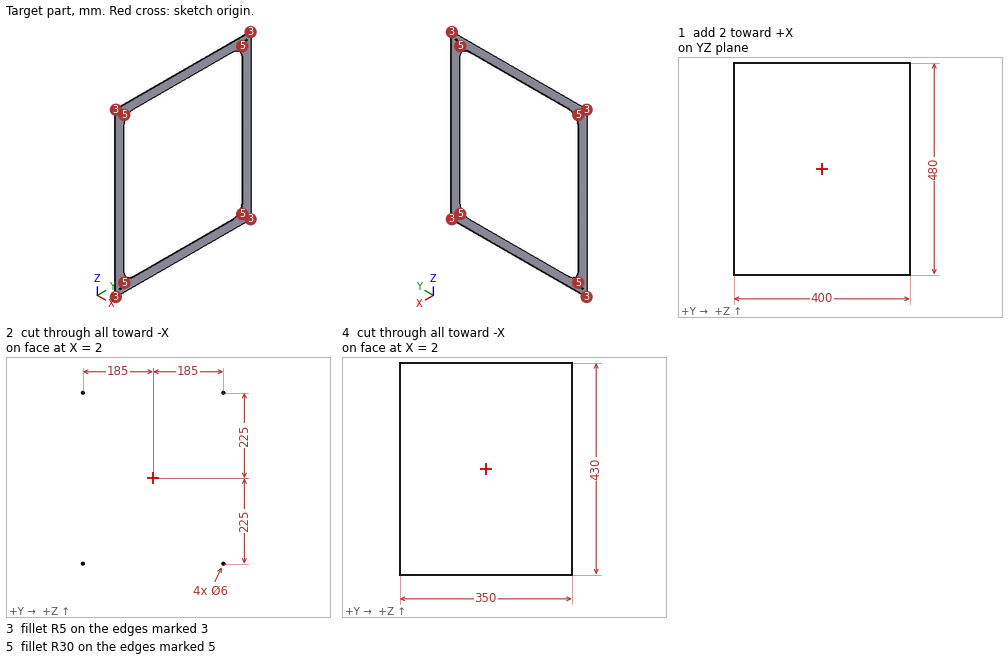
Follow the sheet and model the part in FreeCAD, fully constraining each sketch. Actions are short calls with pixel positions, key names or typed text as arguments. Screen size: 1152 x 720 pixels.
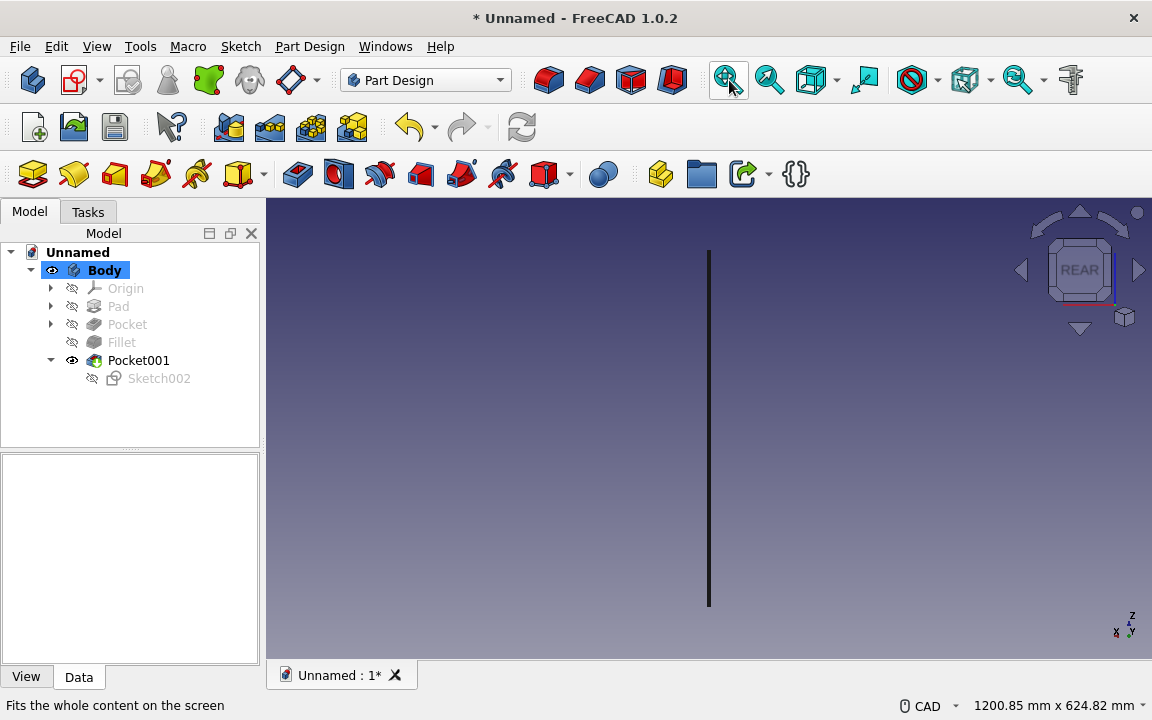
key(6)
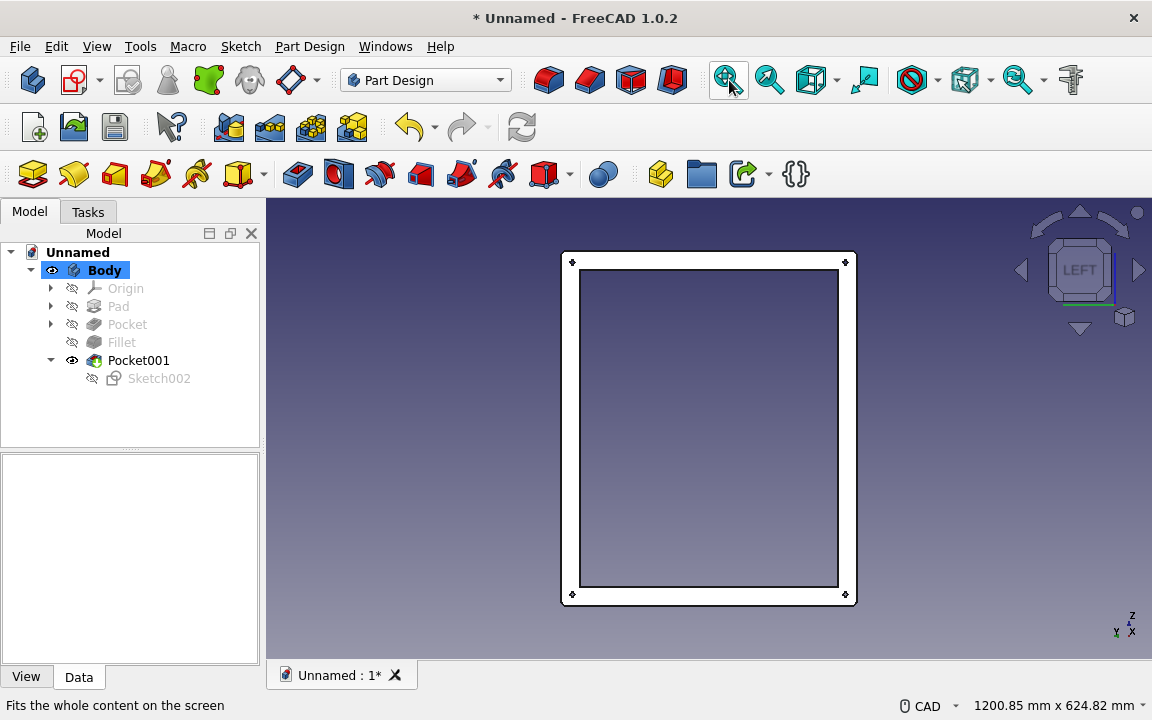
scroll(838, 269, up, 15)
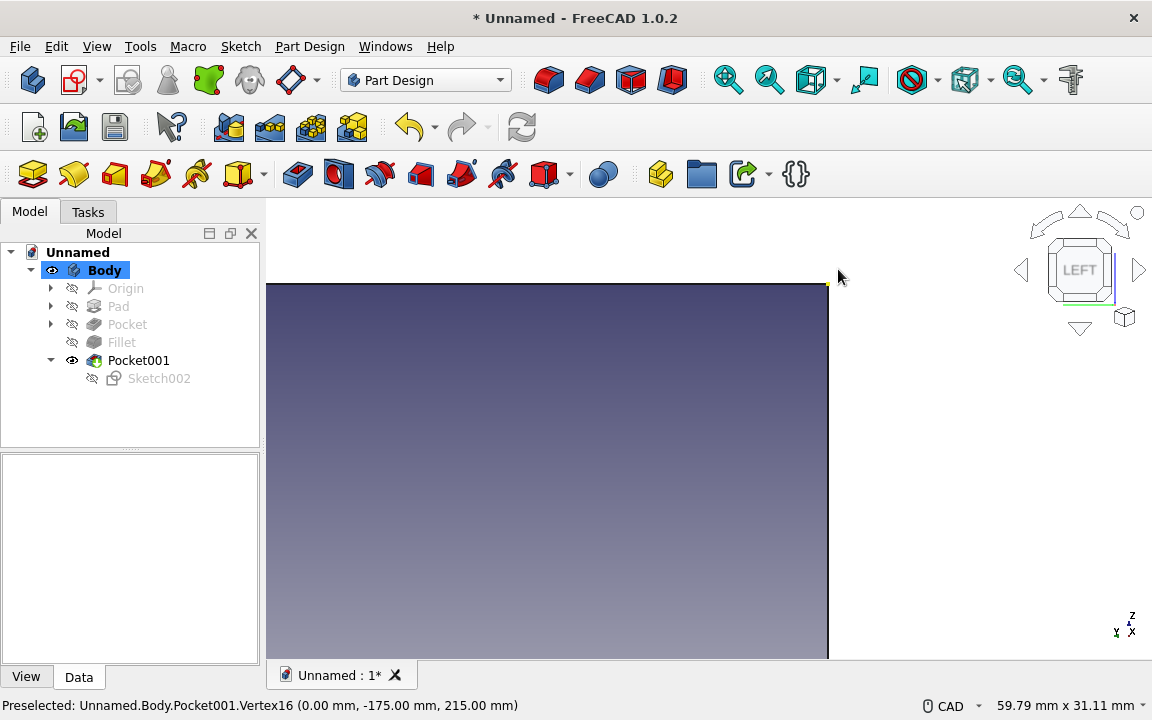
click(729, 80)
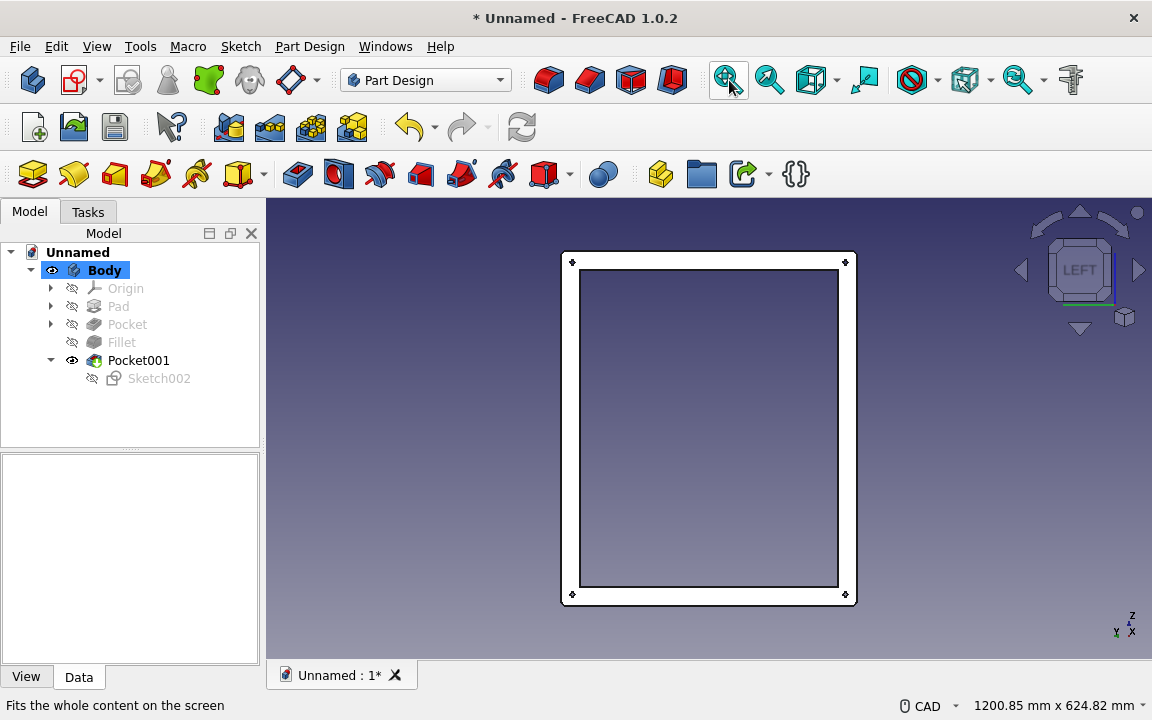
key(v)
key(3)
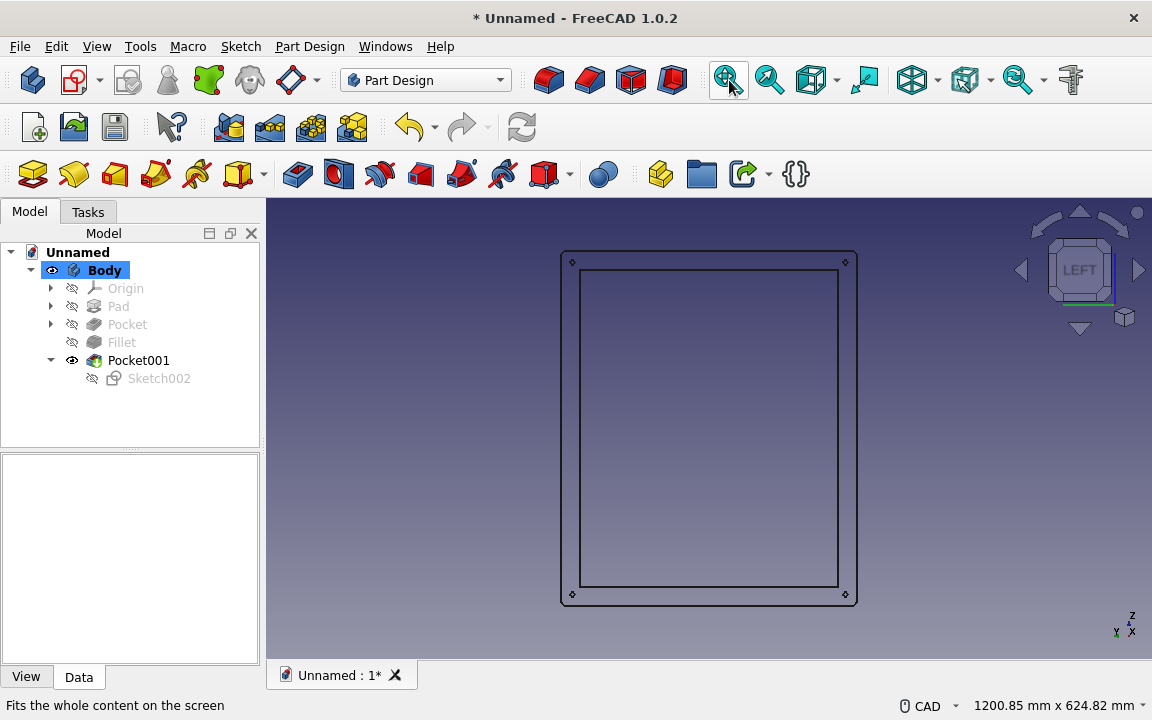
key(0)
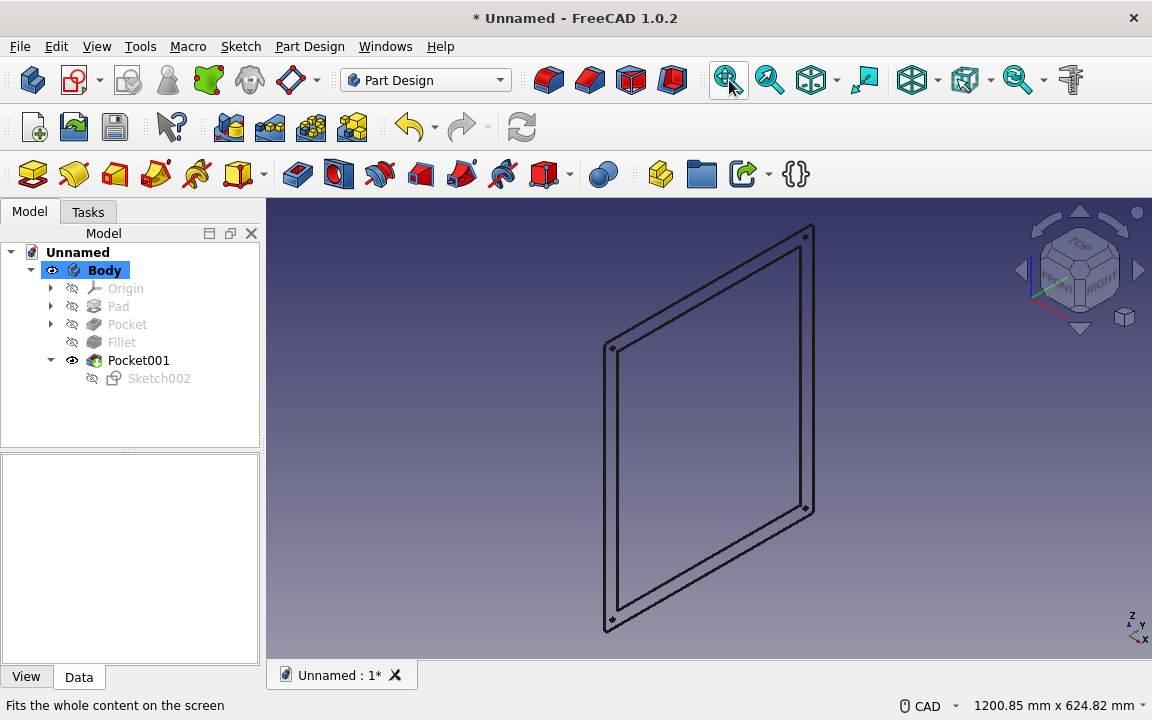
scroll(618, 351, up, 15)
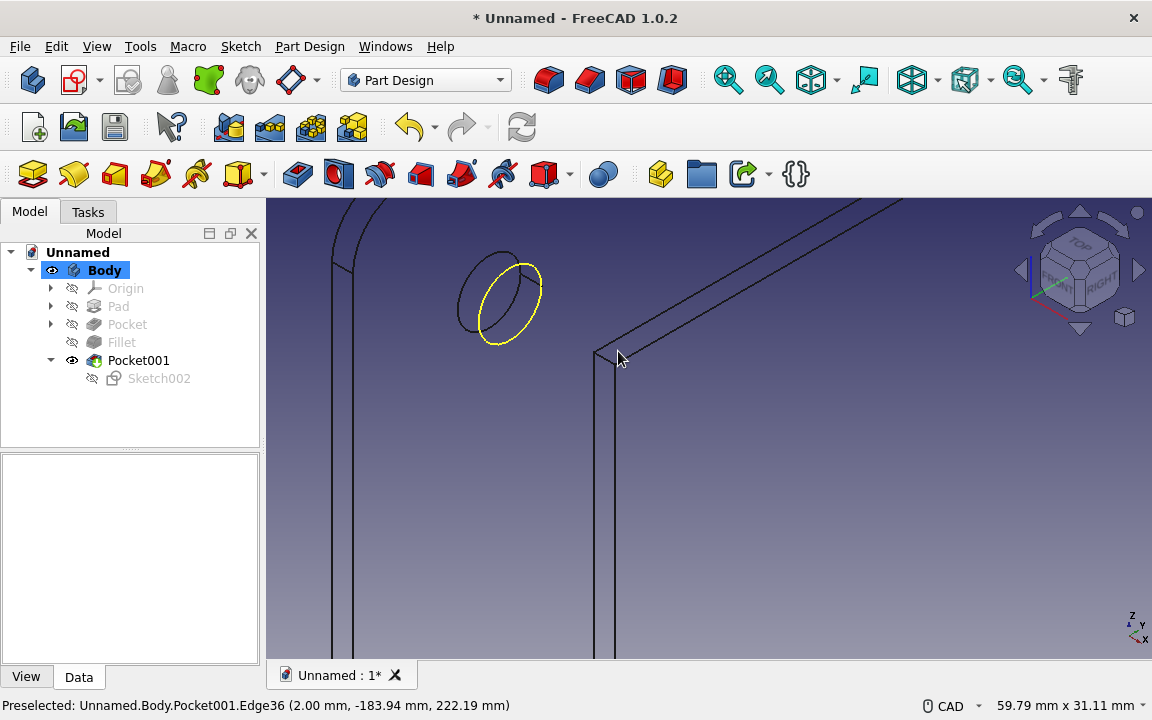
click(604, 358)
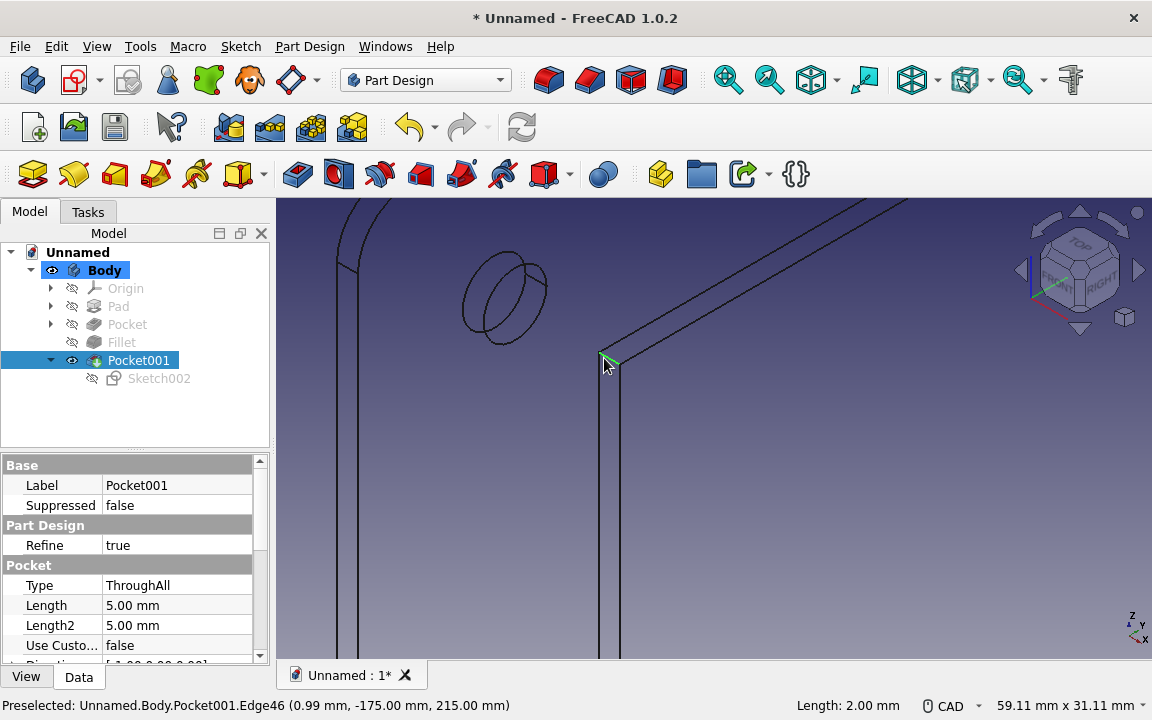
click(729, 80)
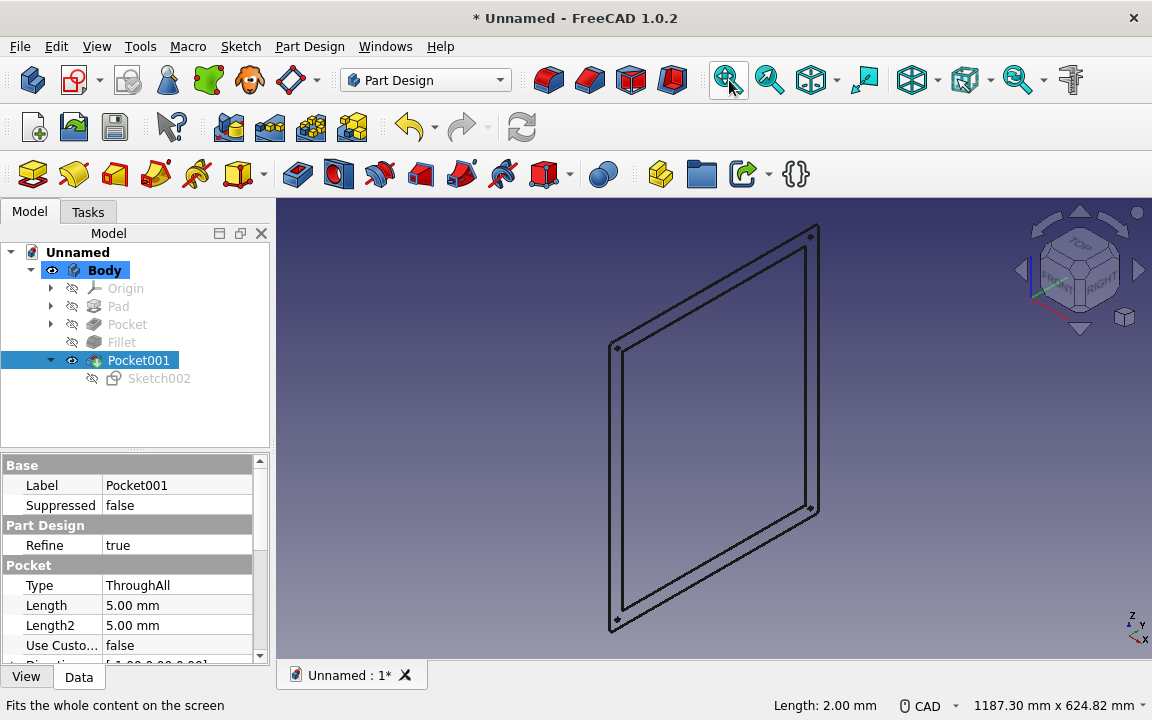
key(2)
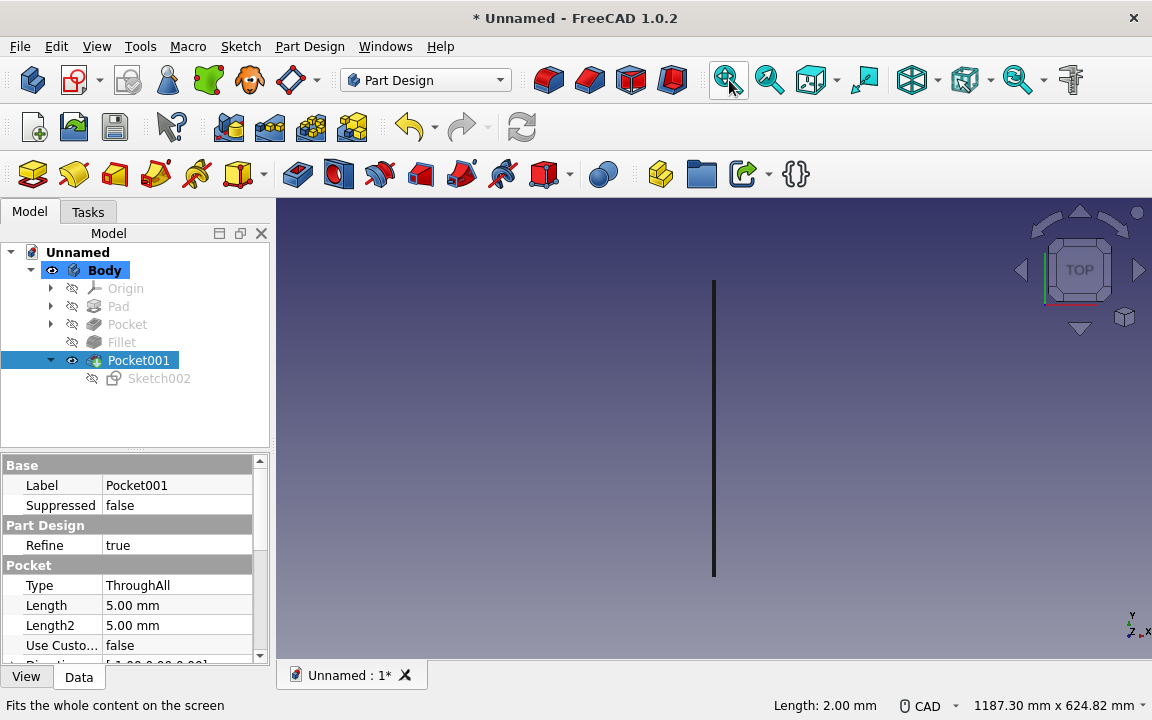
scroll(714, 298, up, 15)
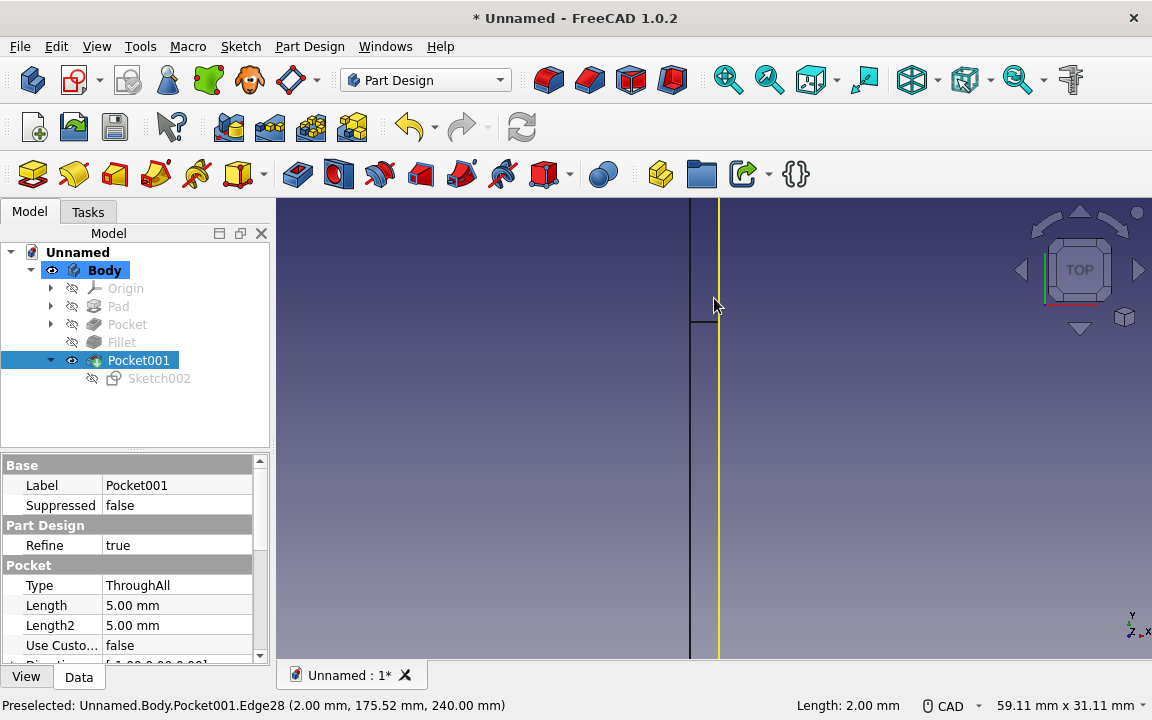
click(704, 321, ctrl)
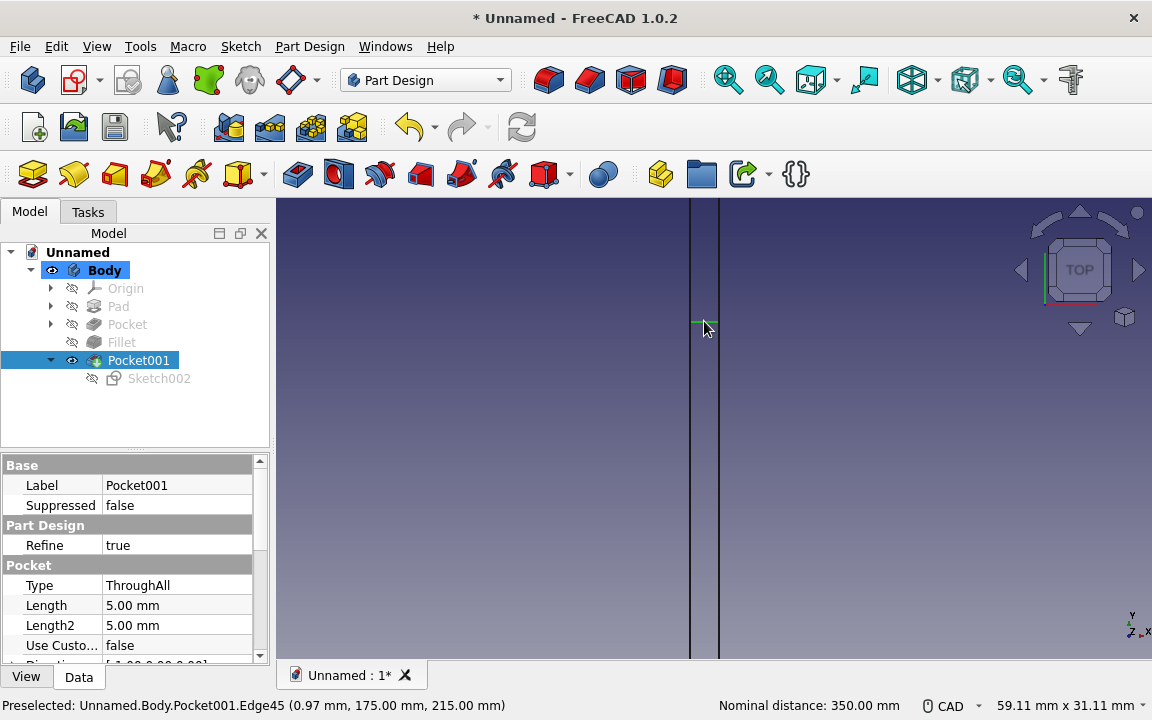
click(729, 80)